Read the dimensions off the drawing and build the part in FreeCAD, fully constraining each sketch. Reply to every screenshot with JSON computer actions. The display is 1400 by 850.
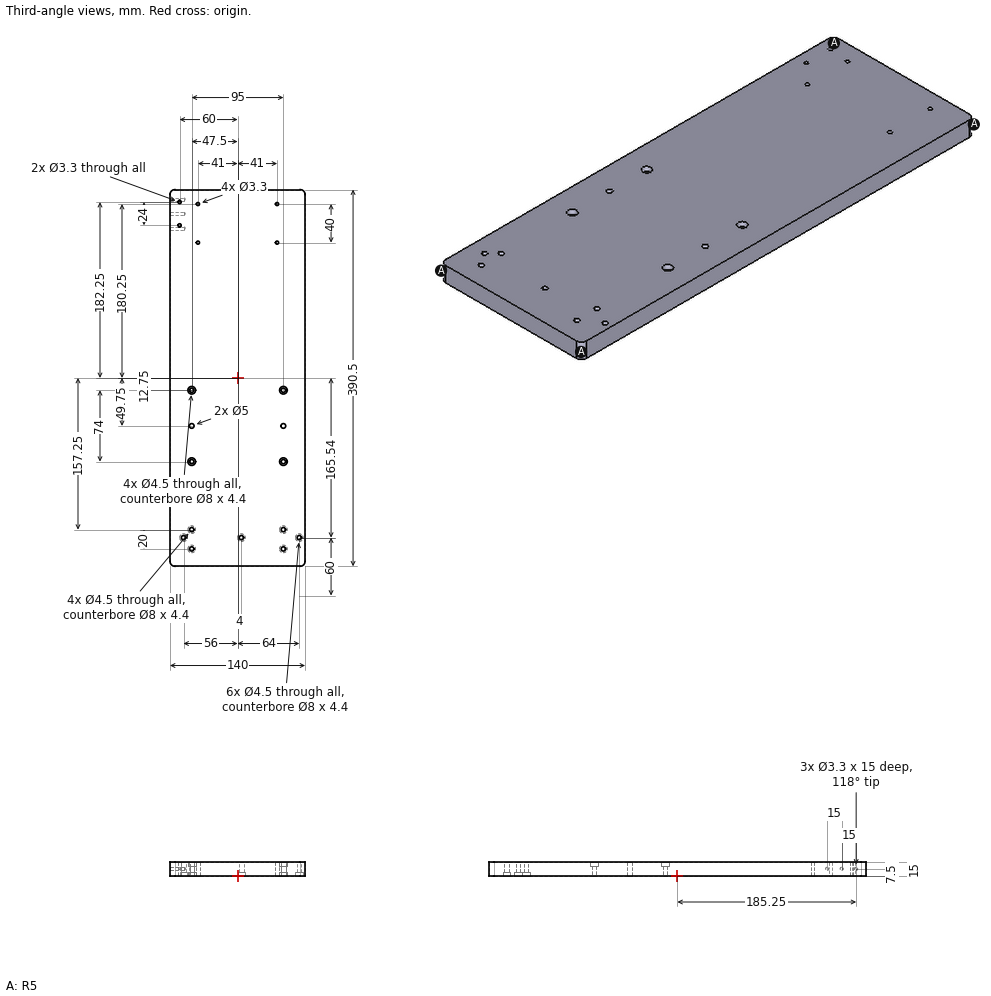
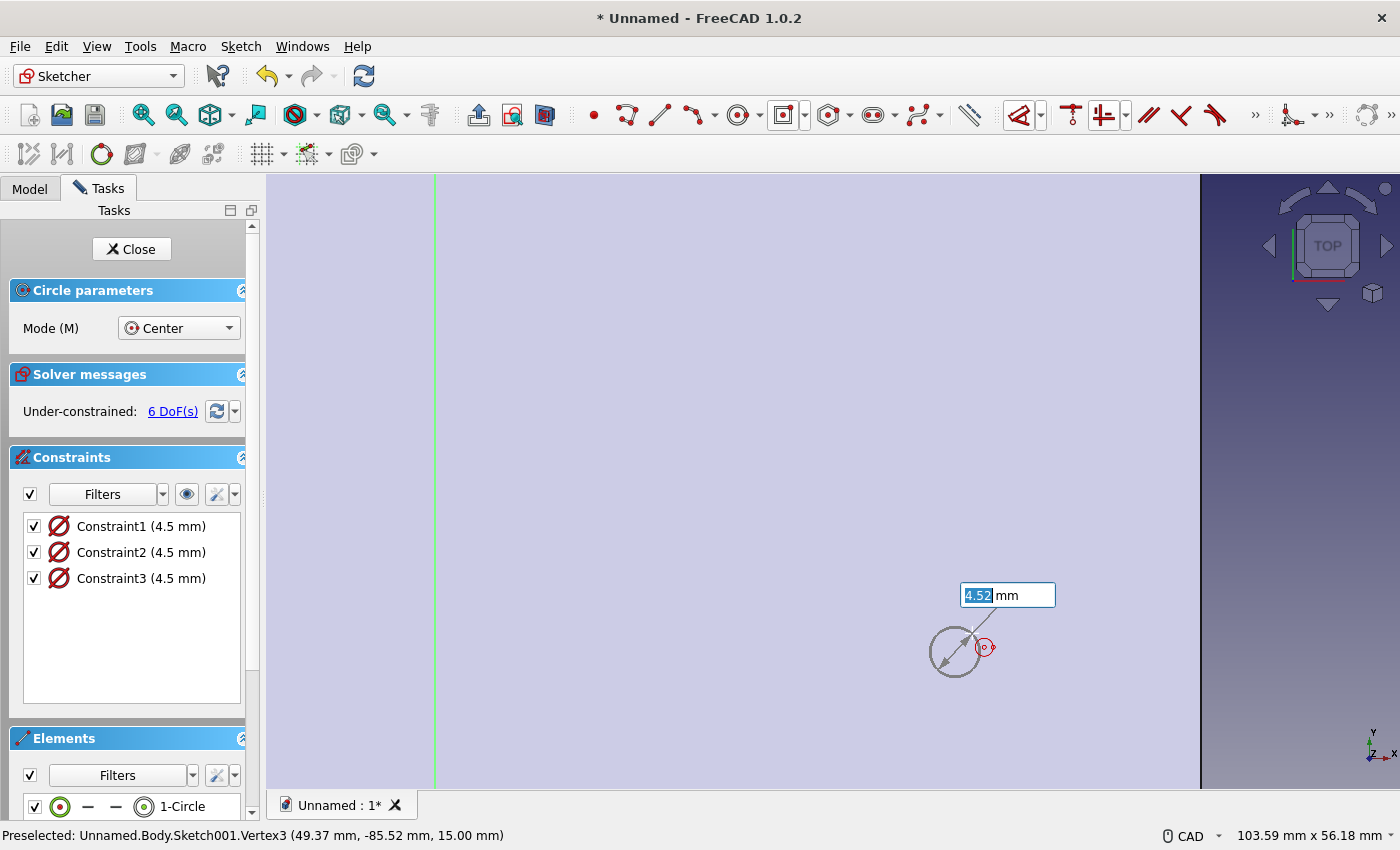
{"action": "type", "text": "4.5"}
{"action": "key", "text": "Return"}
{"action": "key", "text": "Escape"}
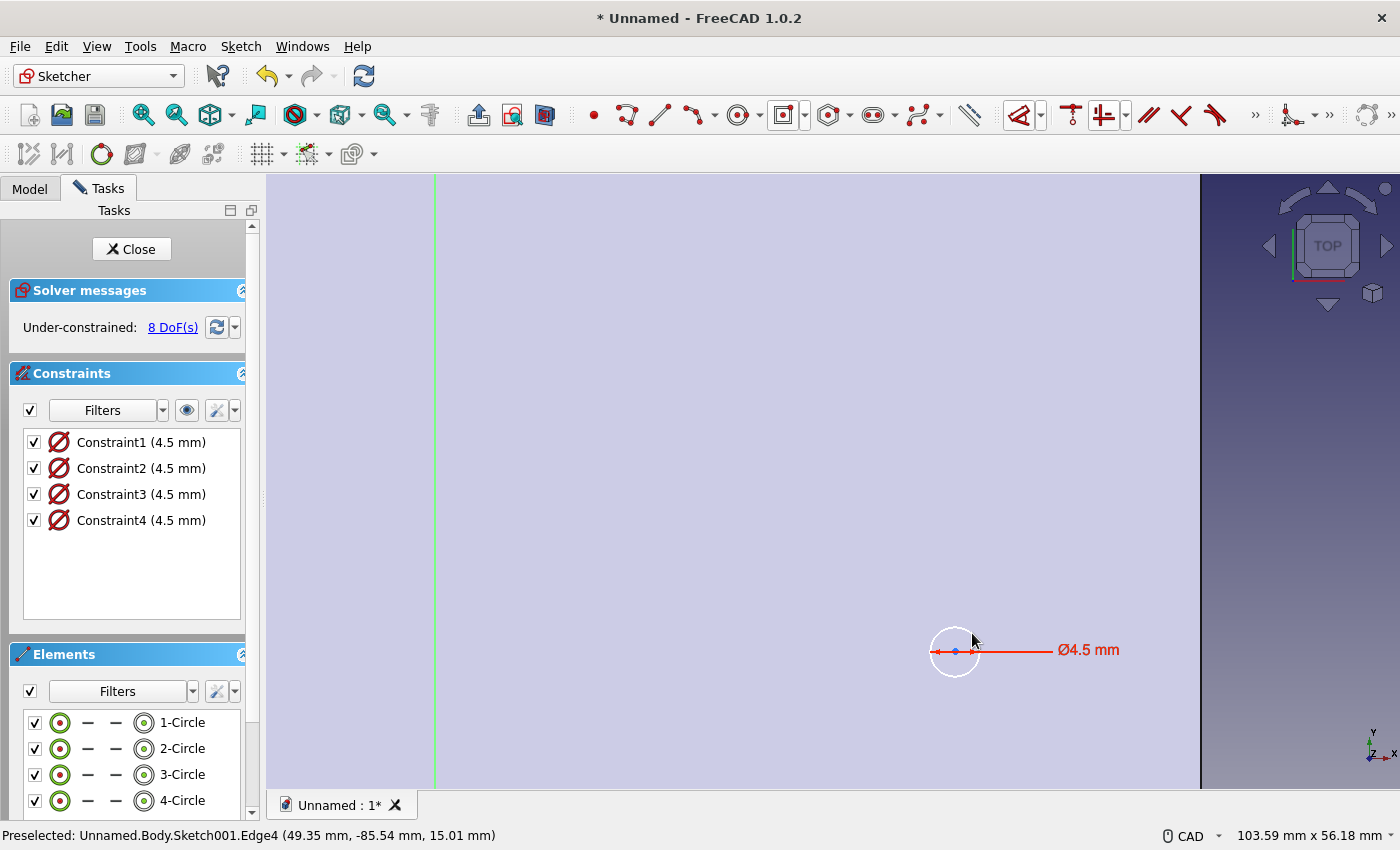
{"action": "scroll", "coordinate": [956, 652], "scroll_direction": "down", "scroll_amount": 5}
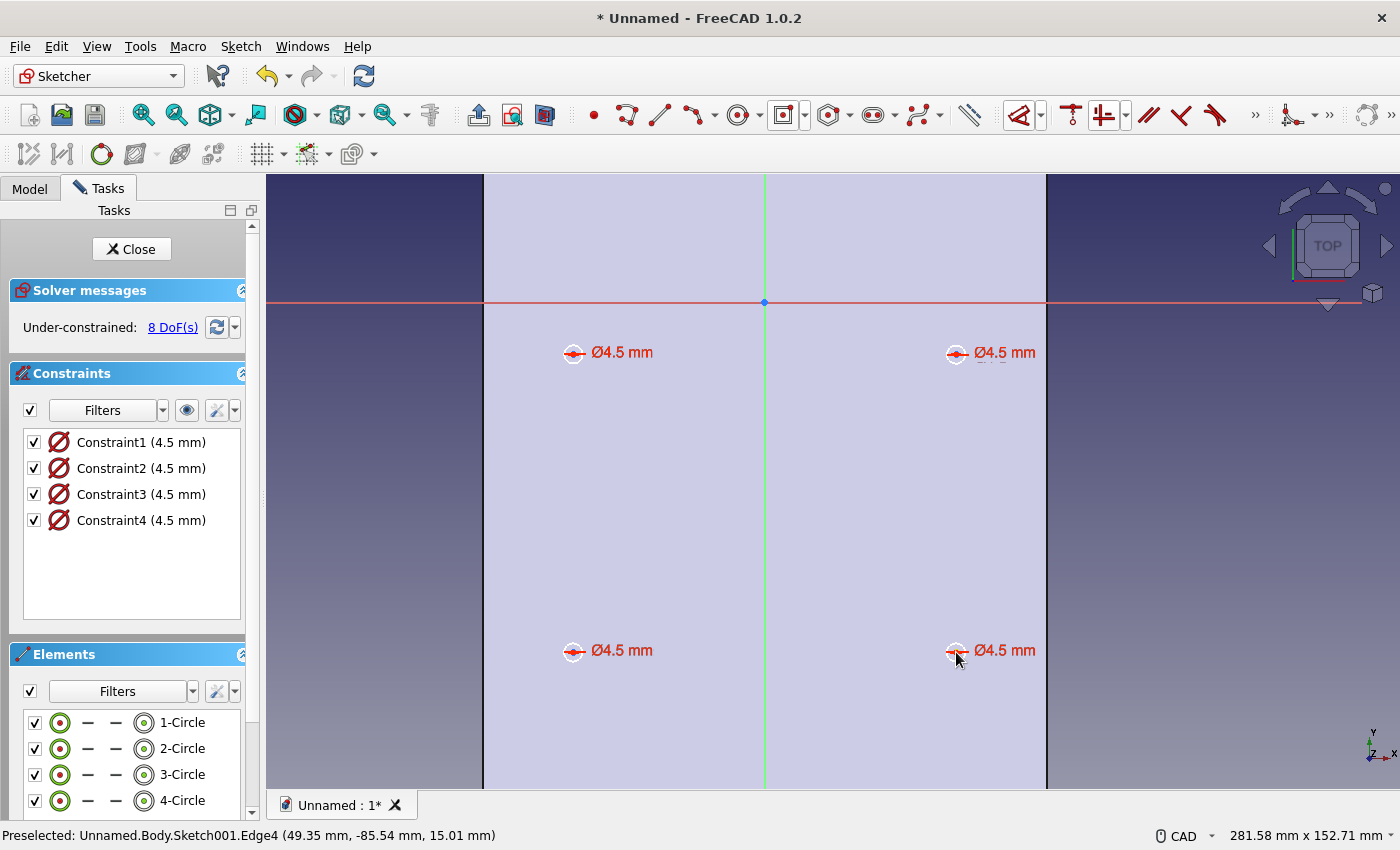
{"action": "left_click", "coordinate": [573, 354]}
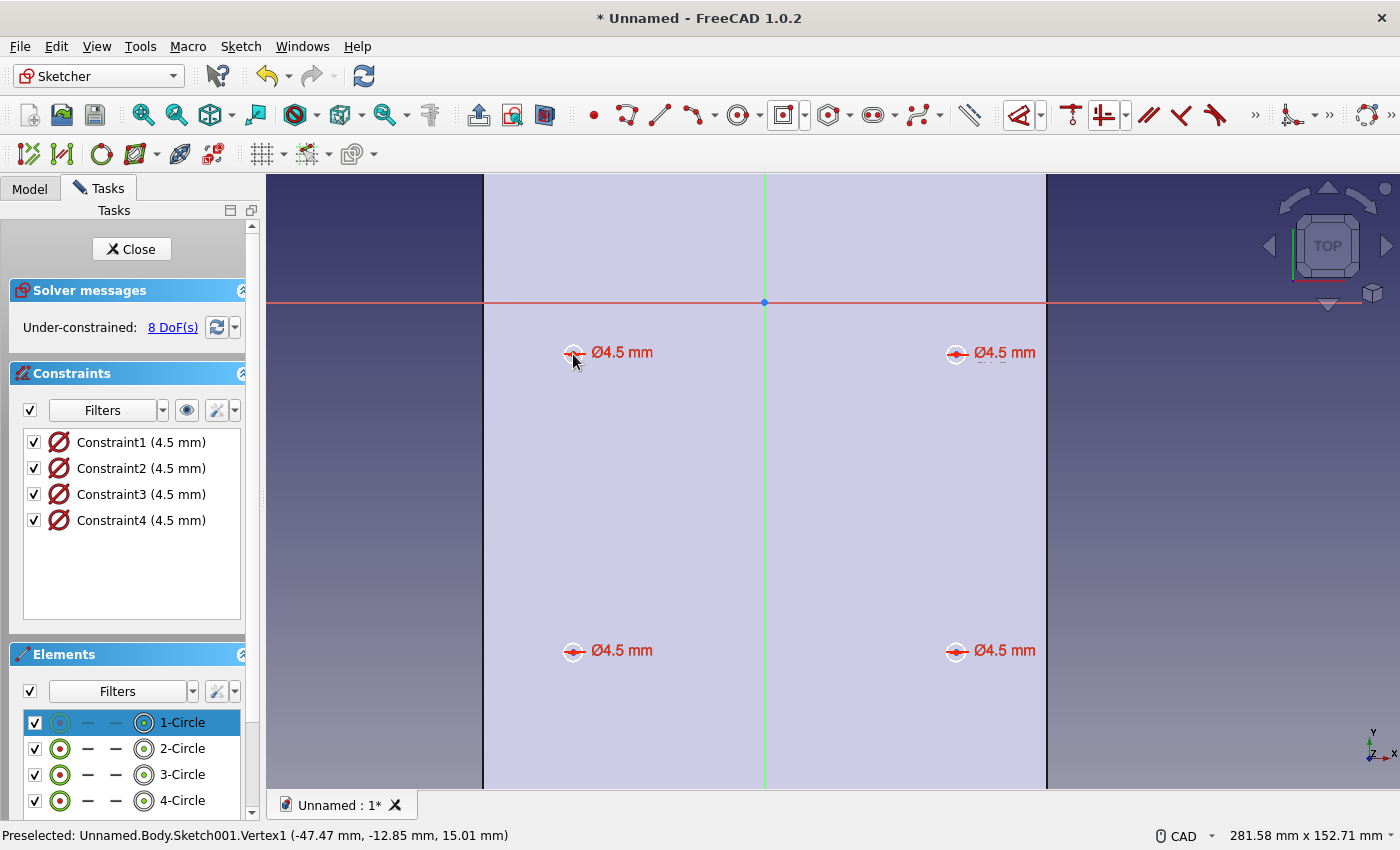
{"action": "left_click", "coordinate": [573, 652]}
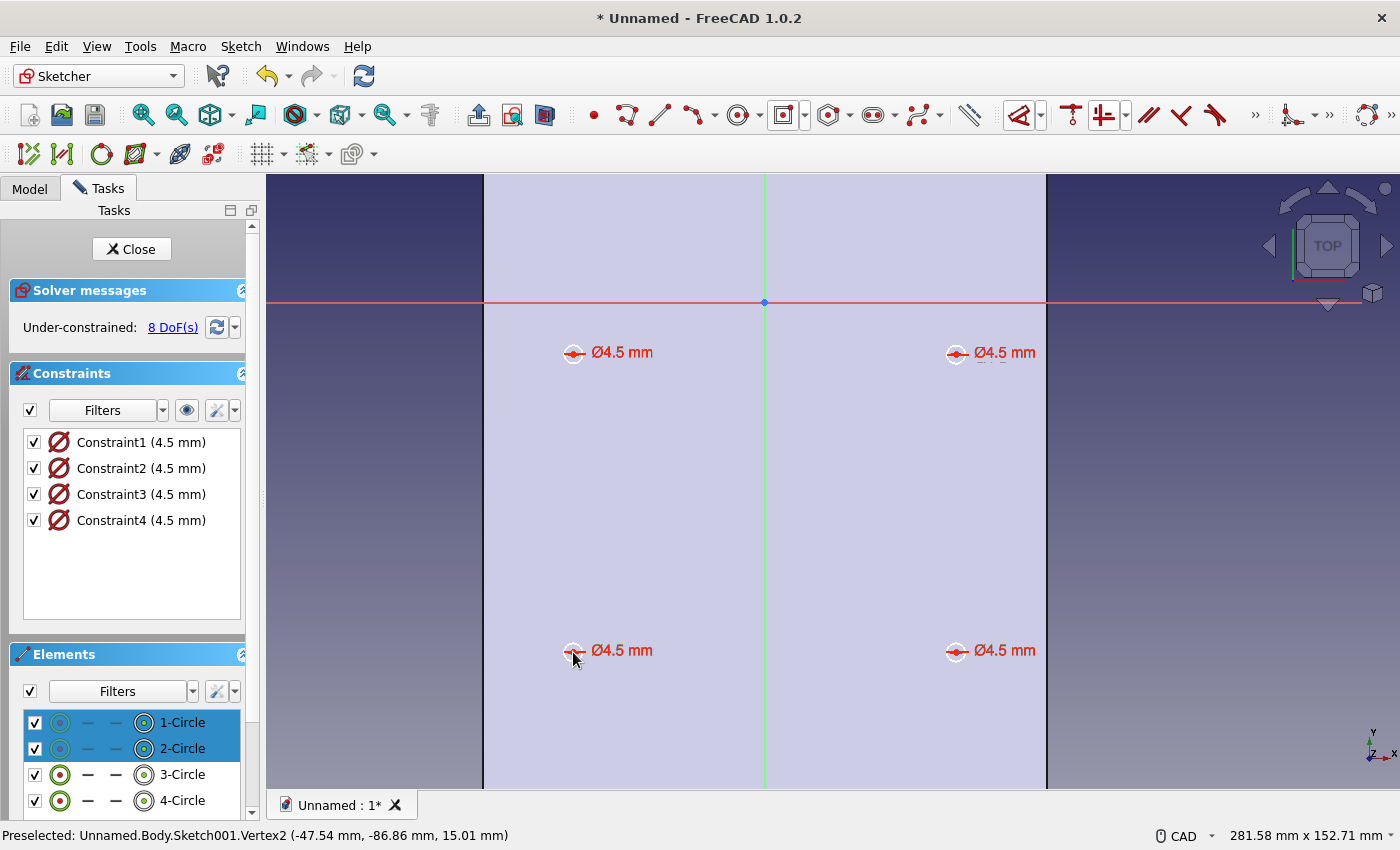
{"action": "left_click", "coordinate": [1126, 116]}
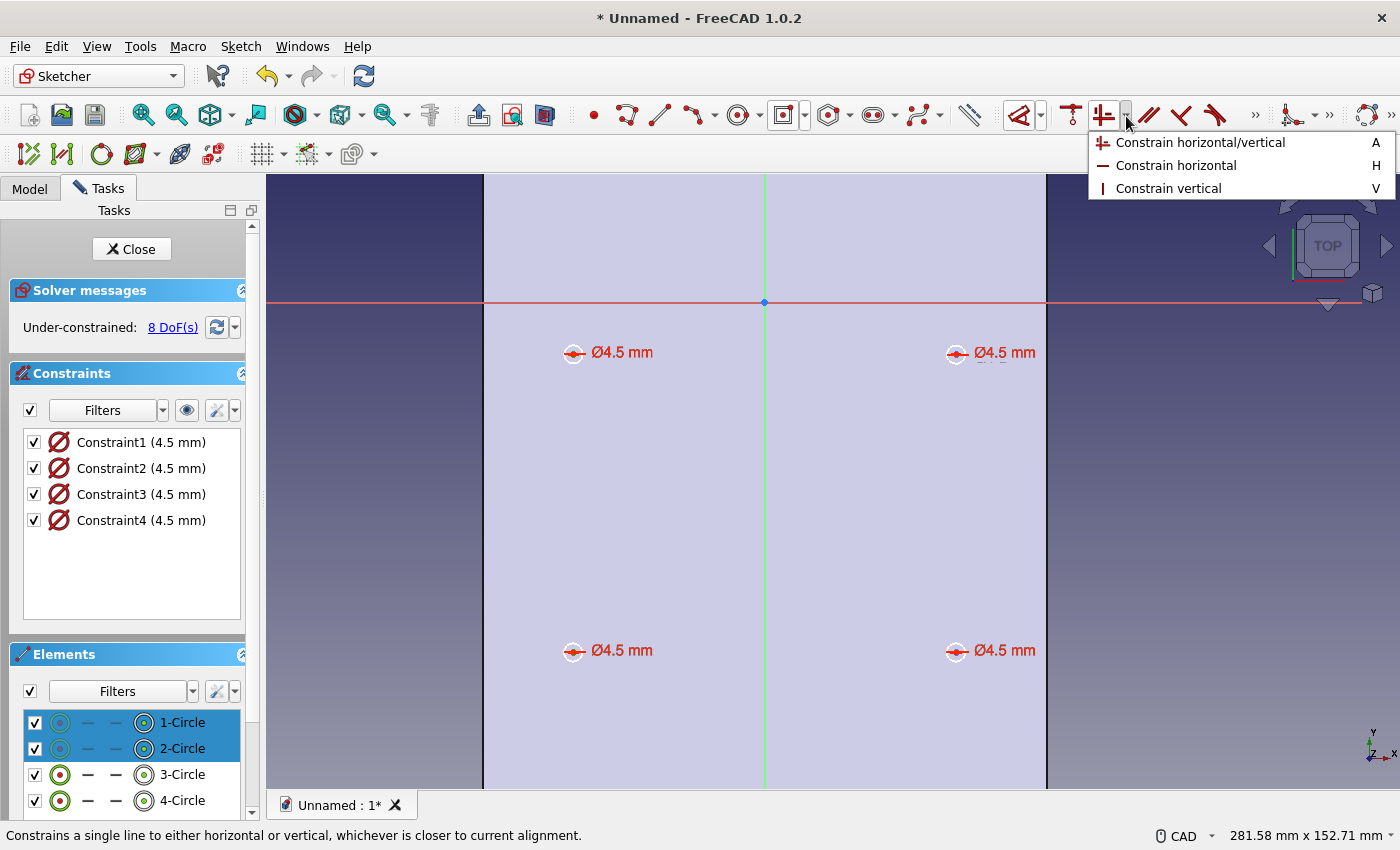
{"action": "left_click", "coordinate": [1242, 188]}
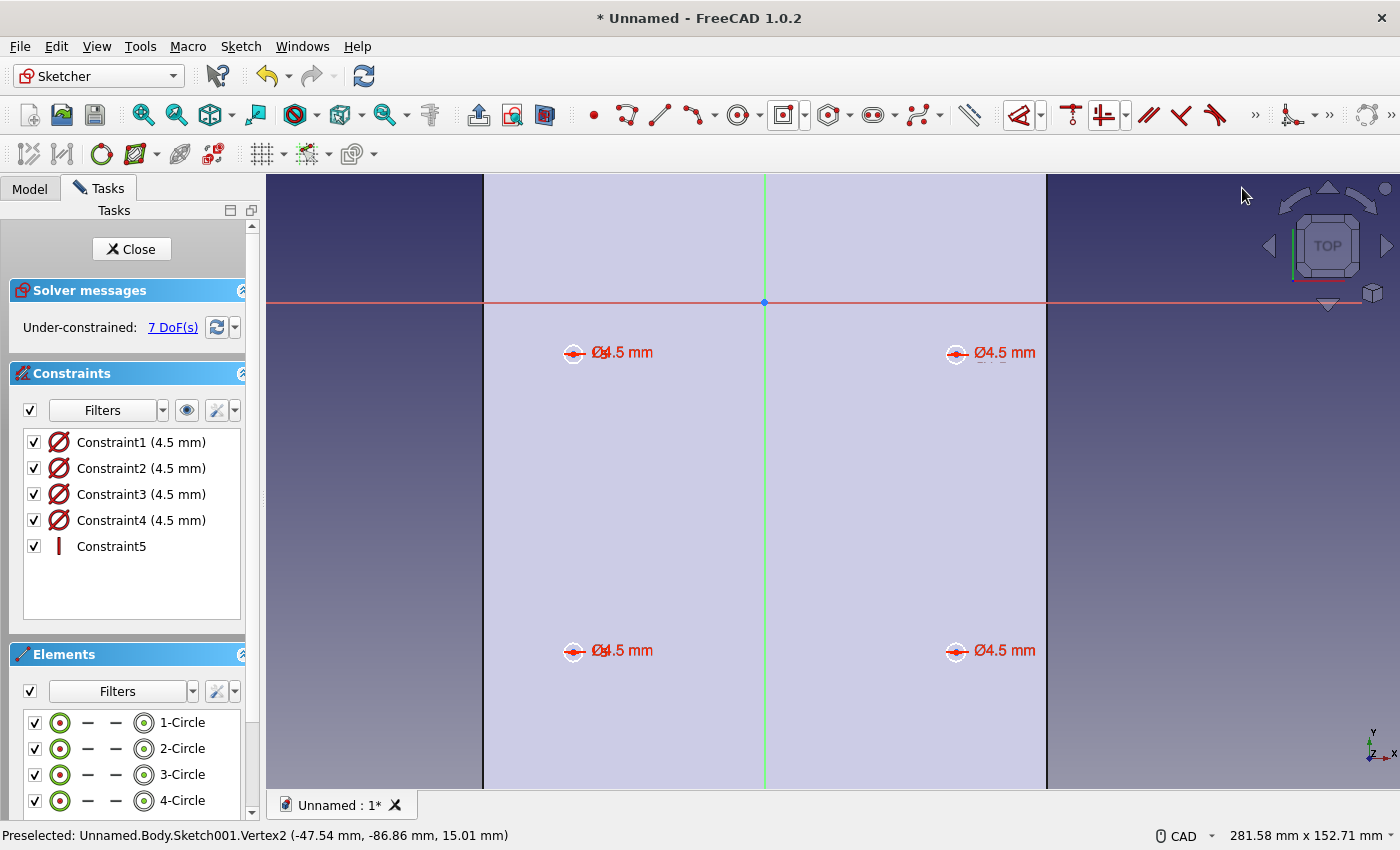
{"action": "left_click", "coordinate": [573, 354]}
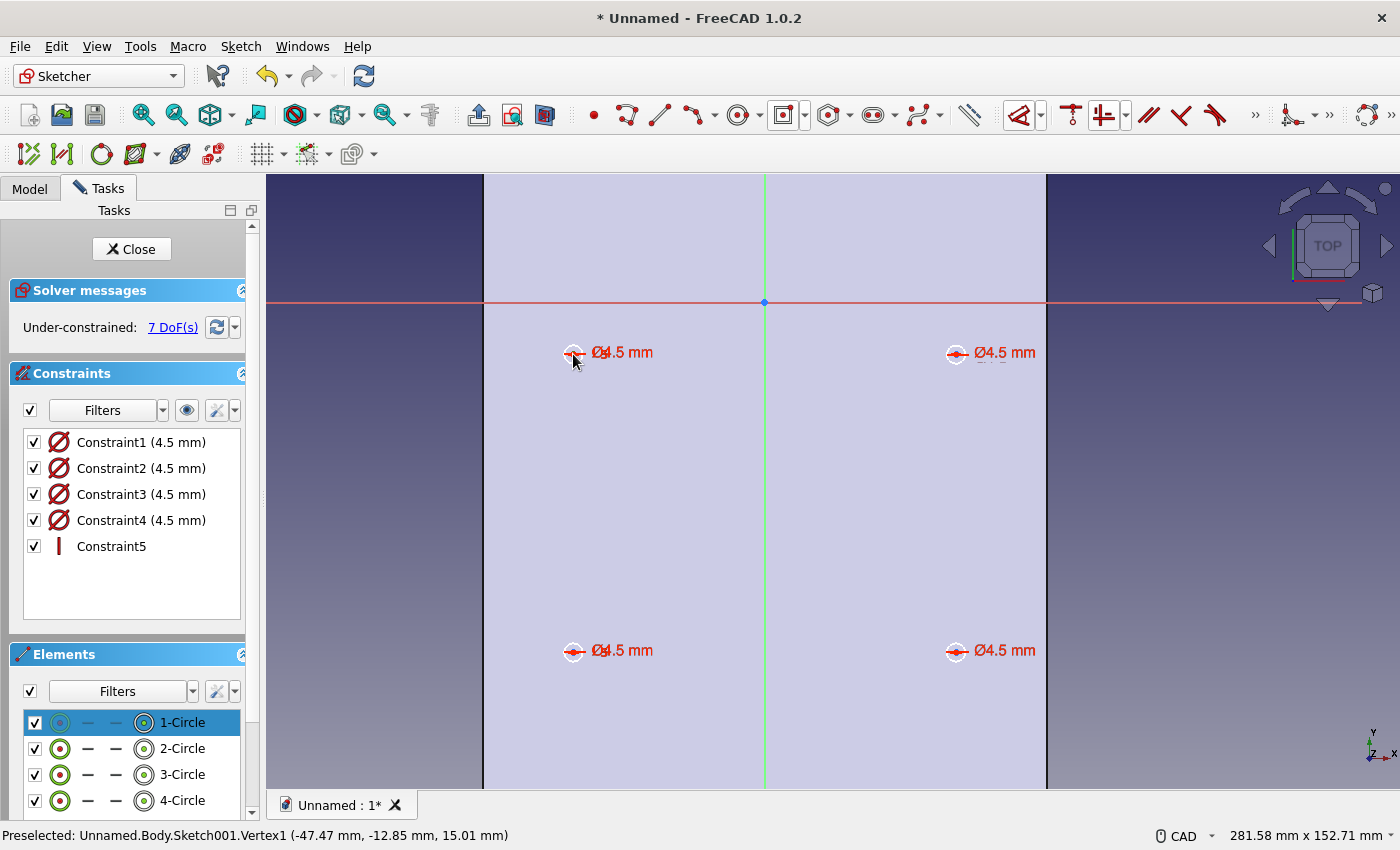
{"action": "left_click", "coordinate": [956, 355]}